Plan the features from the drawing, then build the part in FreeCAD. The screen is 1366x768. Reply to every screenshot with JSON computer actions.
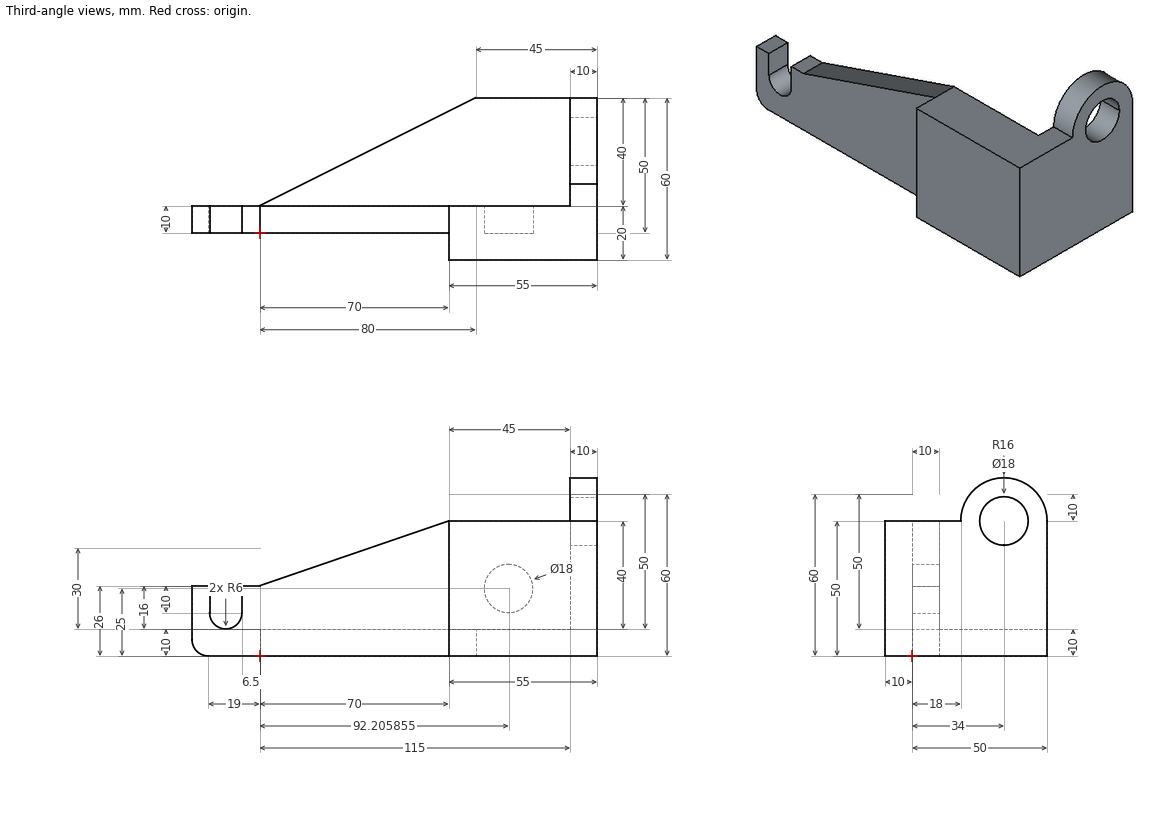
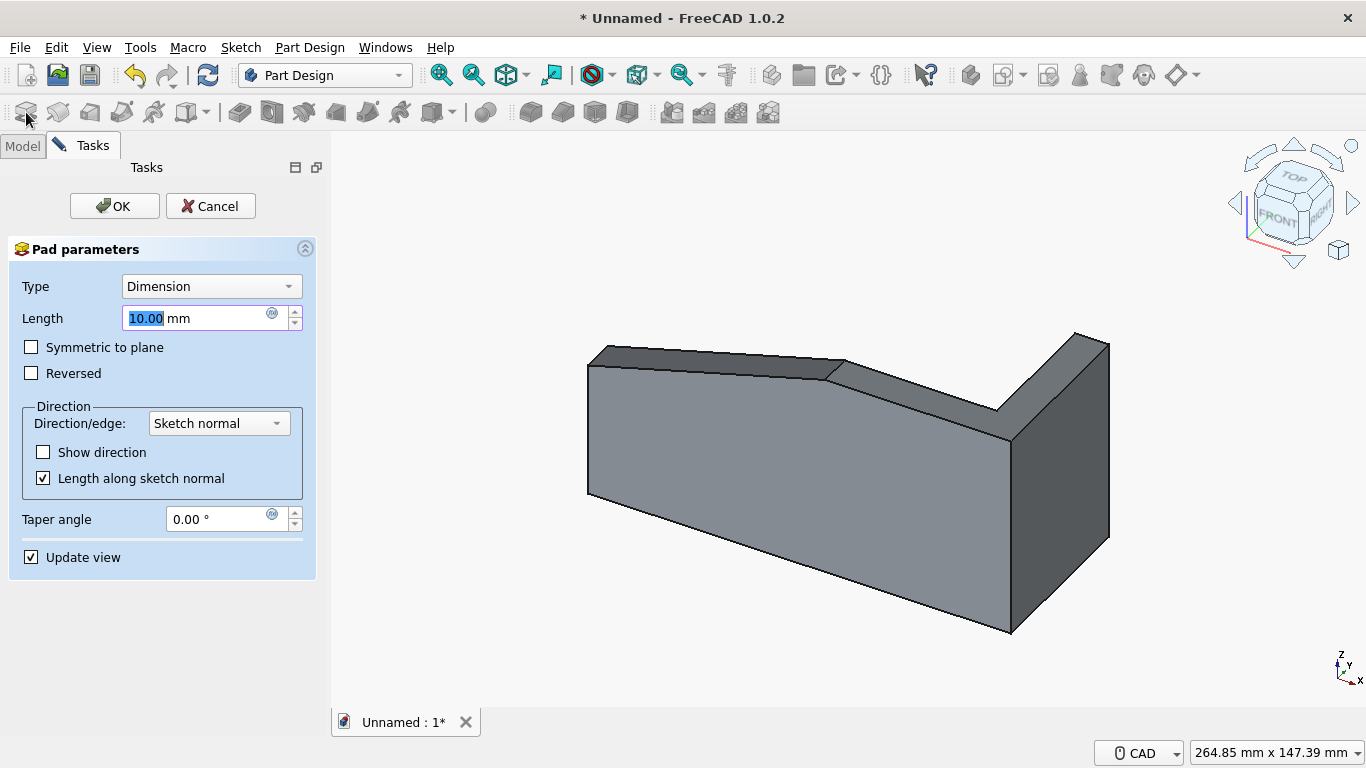
{"action": "type", "text": "10"}
{"action": "key", "text": "Tab"}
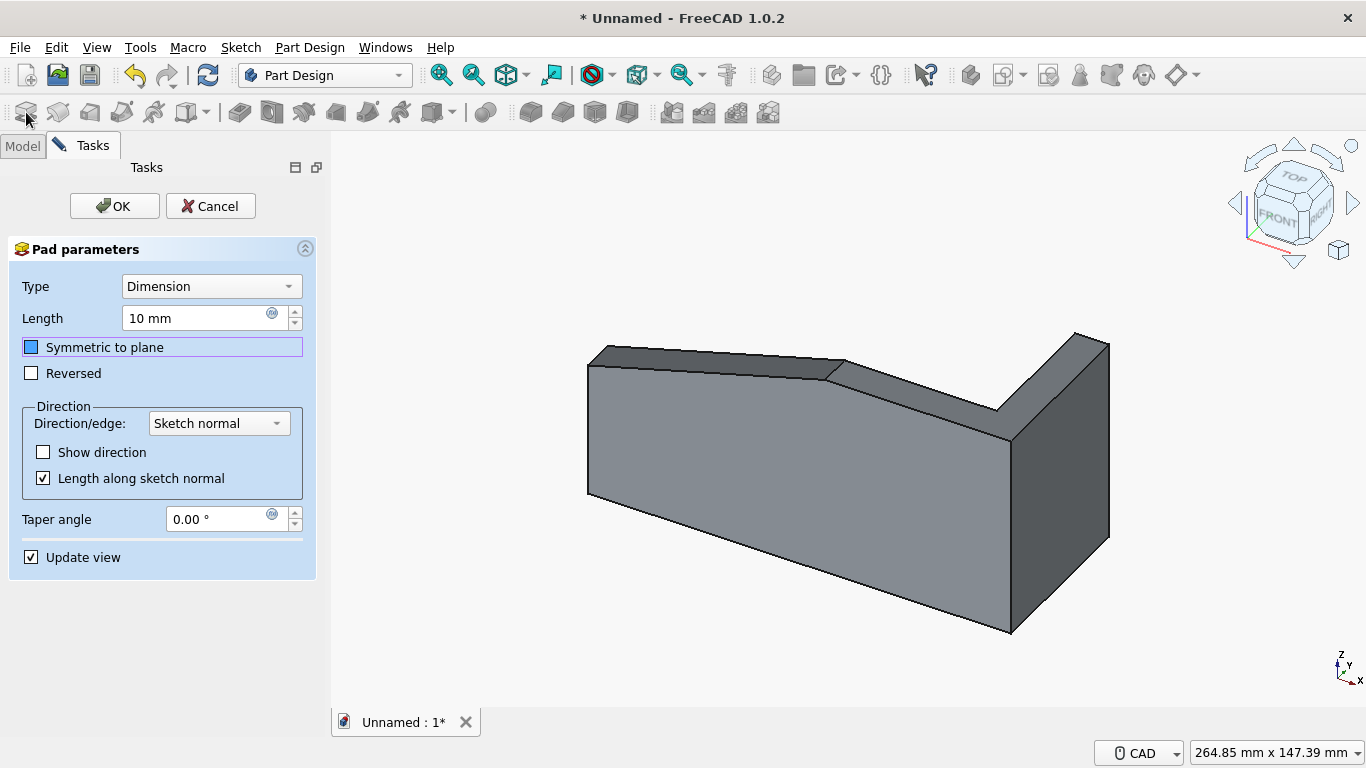
{"action": "left_click", "coordinate": [115, 206]}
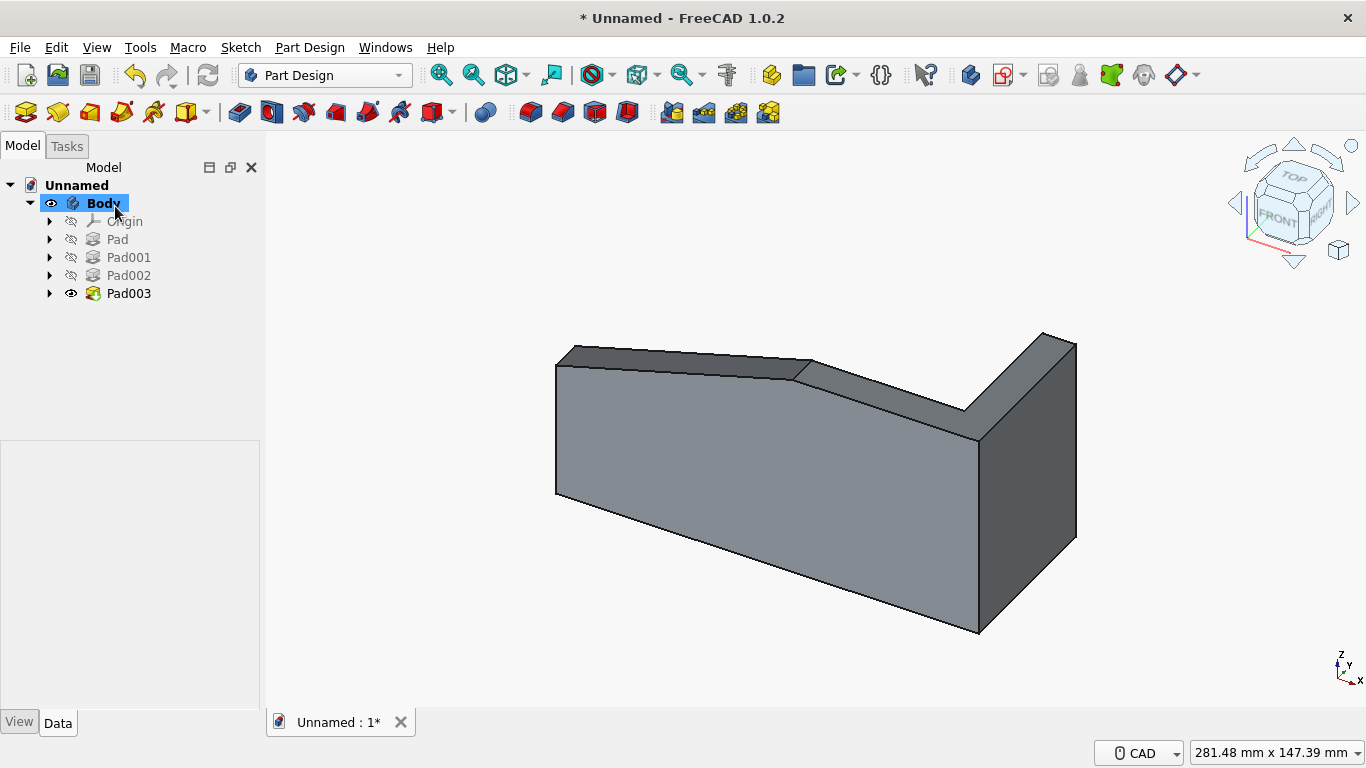
{"action": "left_click", "coordinate": [828, 487]}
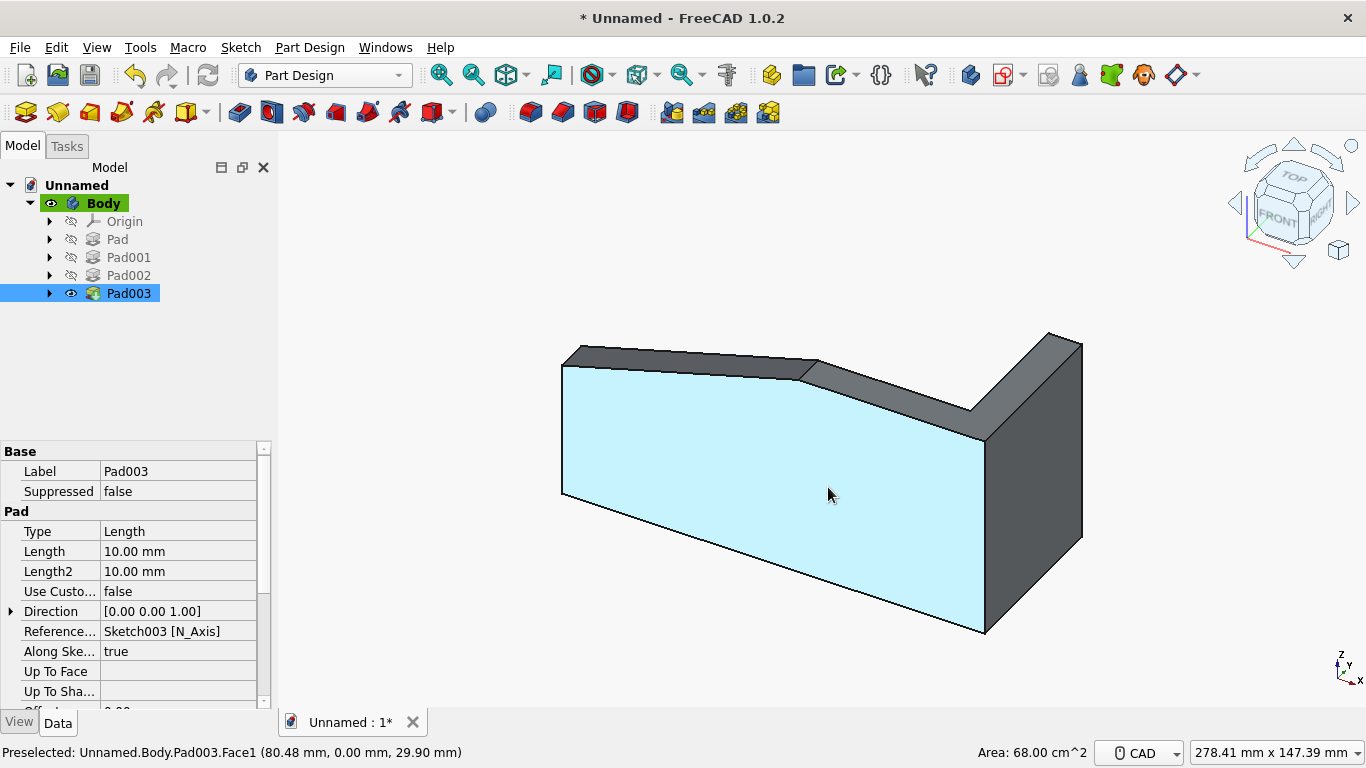
{"action": "left_click", "coordinate": [1004, 76]}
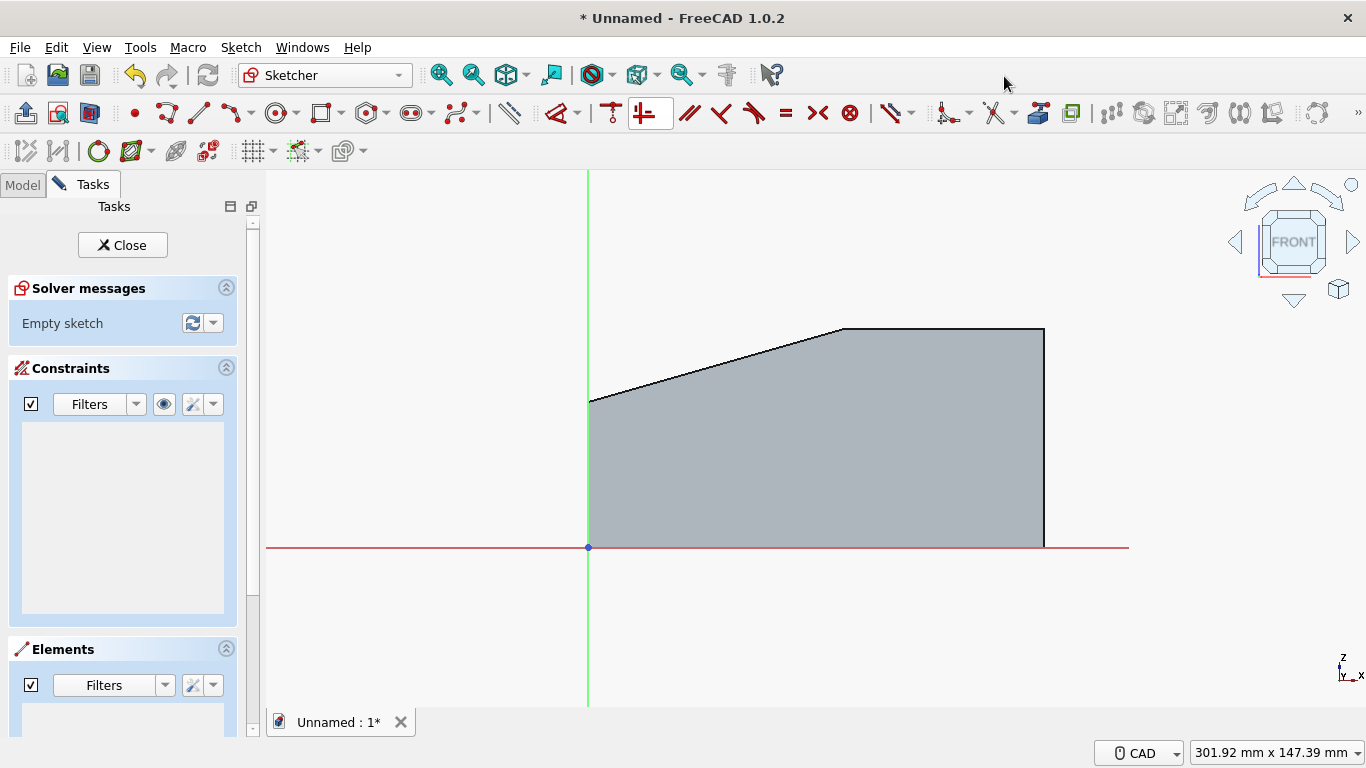
{"action": "scroll", "coordinate": [955, 439], "scroll_direction": "up", "scroll_amount": 2}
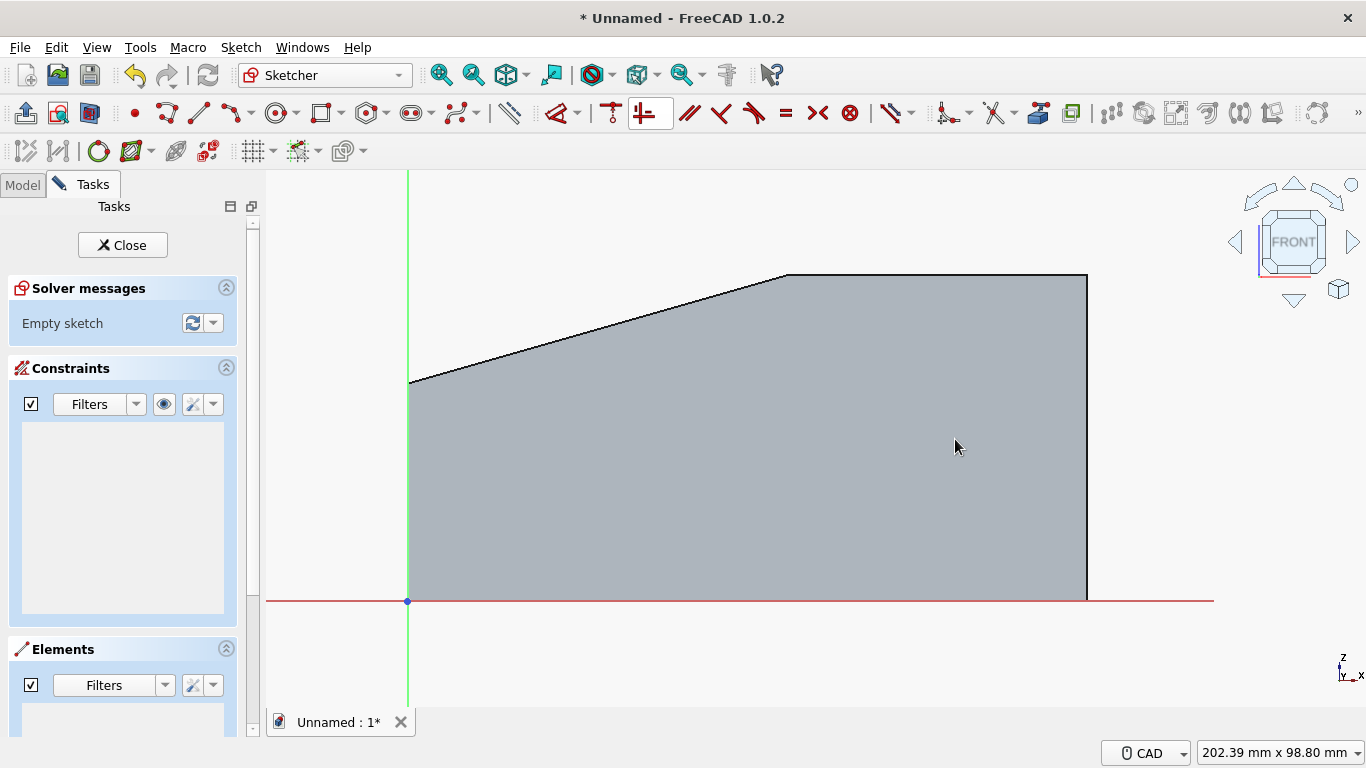
{"action": "left_click", "coordinate": [322, 114]}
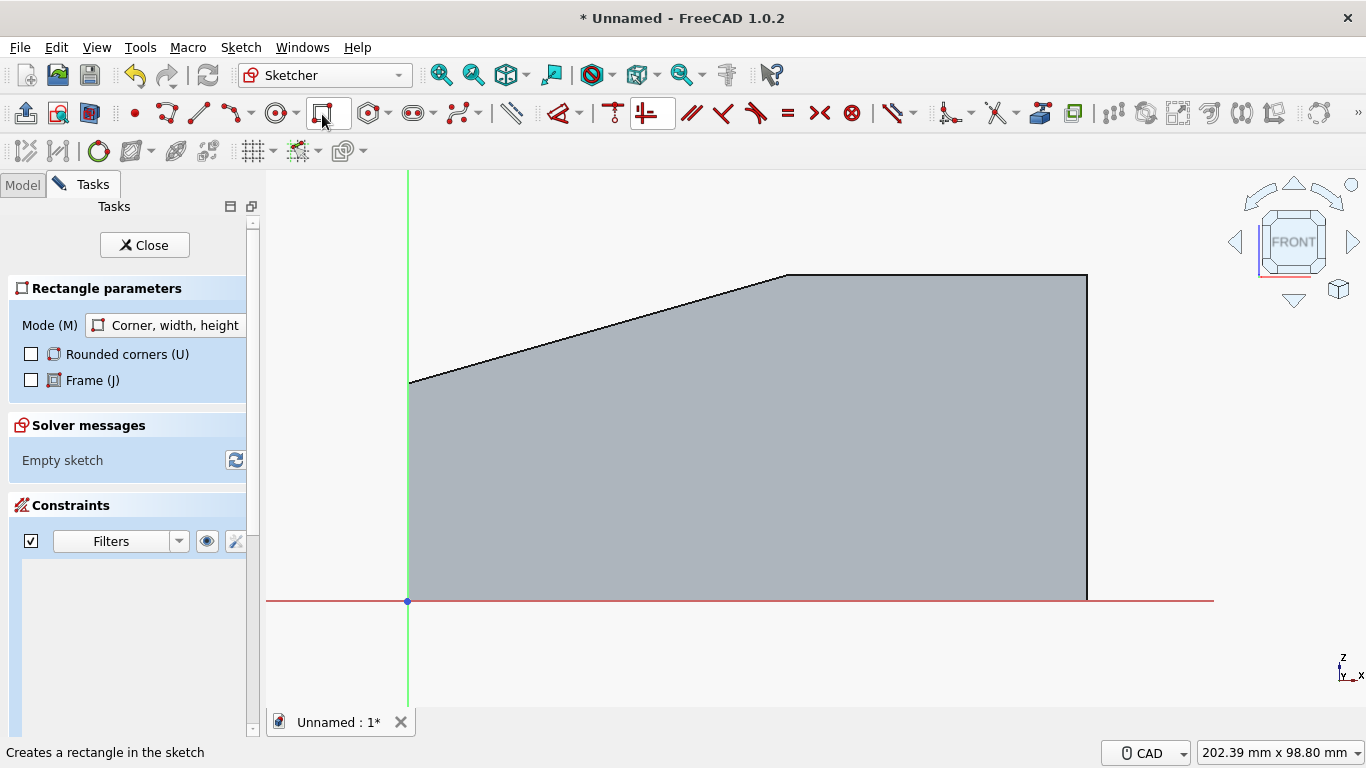
{"action": "left_click", "coordinate": [788, 275]}
{"action": "left_click", "coordinate": [1087, 601]}
{"action": "key", "text": "Escape"}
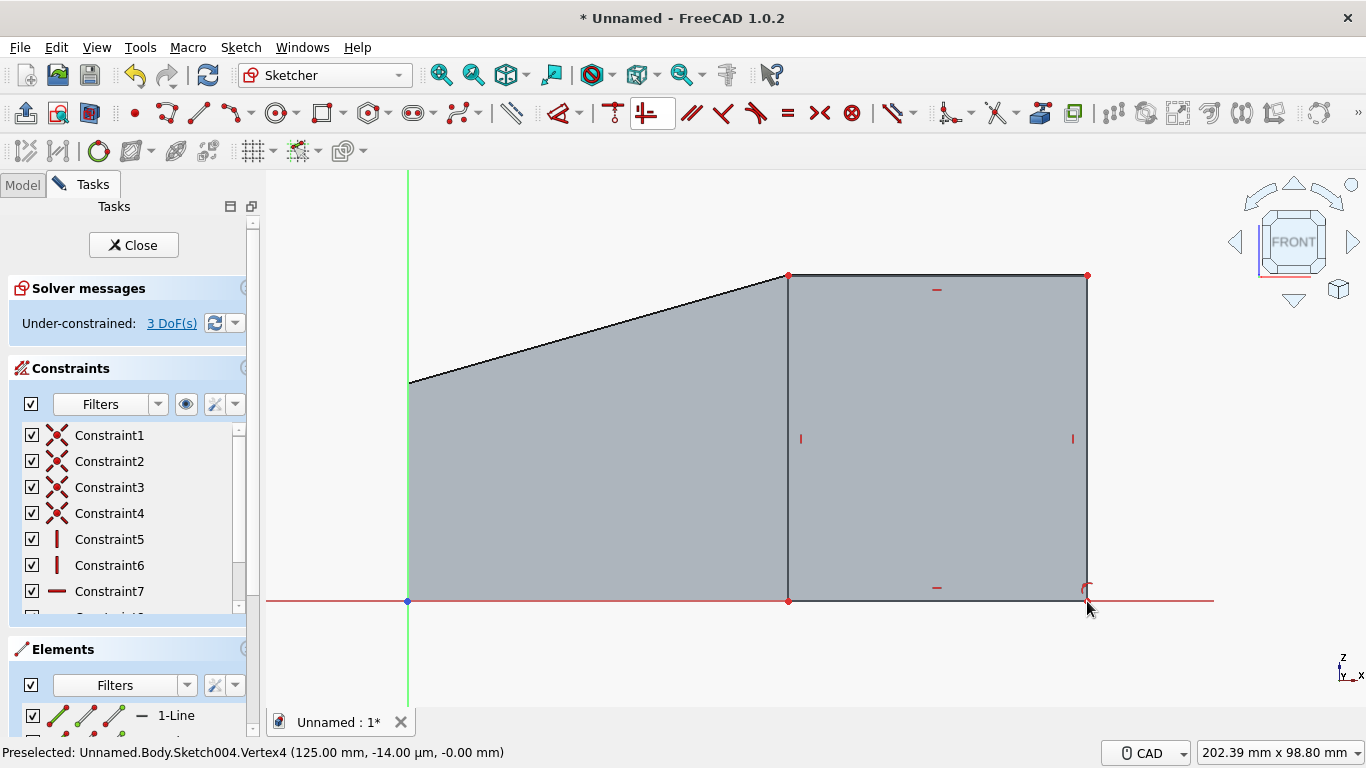
{"action": "left_click", "coordinate": [558, 114]}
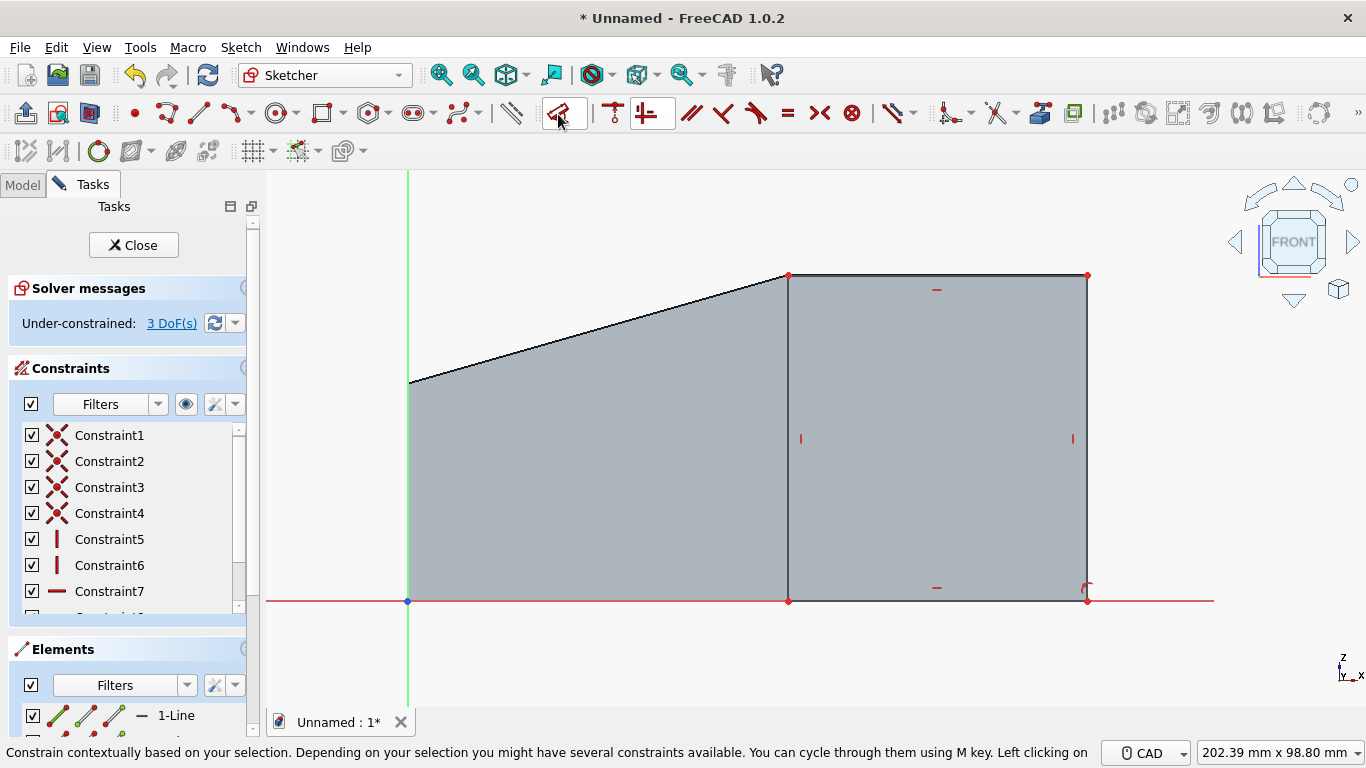
{"action": "left_click", "coordinate": [788, 374]}
{"action": "left_click", "coordinate": [822, 439]}